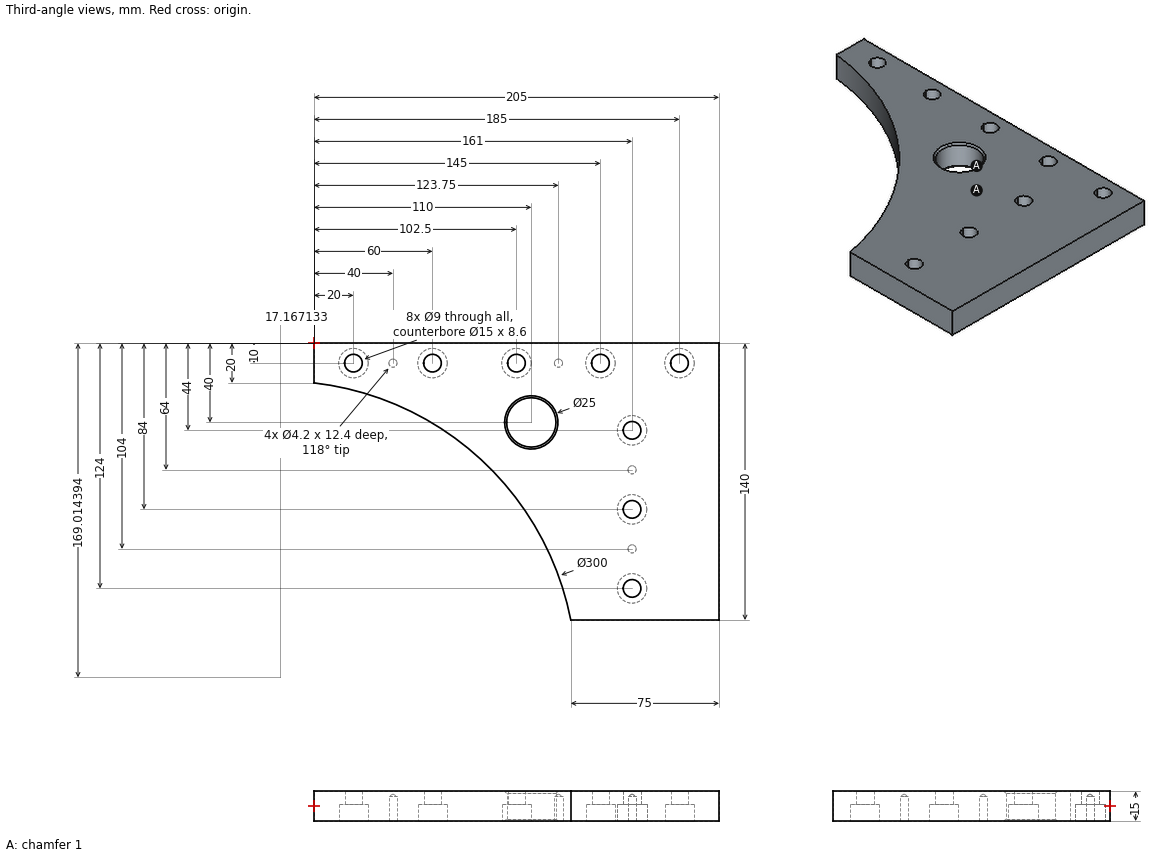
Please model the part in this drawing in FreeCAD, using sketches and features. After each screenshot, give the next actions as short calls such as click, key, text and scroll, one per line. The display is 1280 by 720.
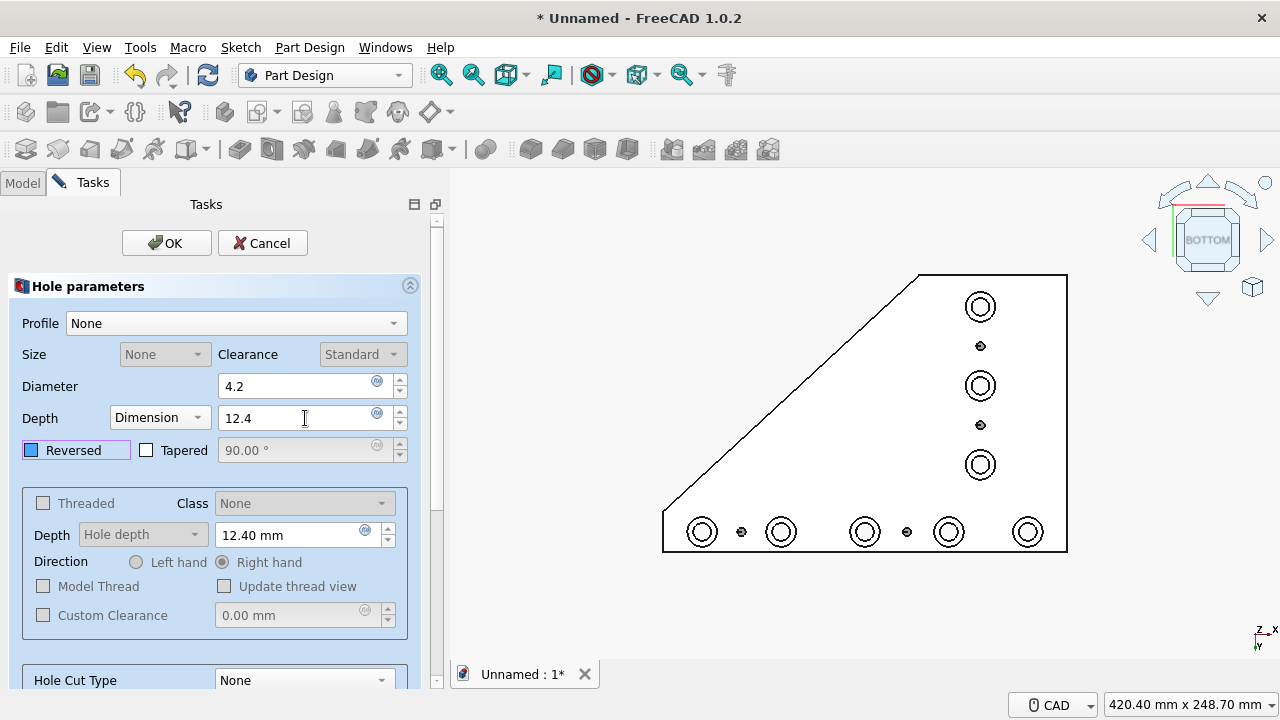
click(167, 243)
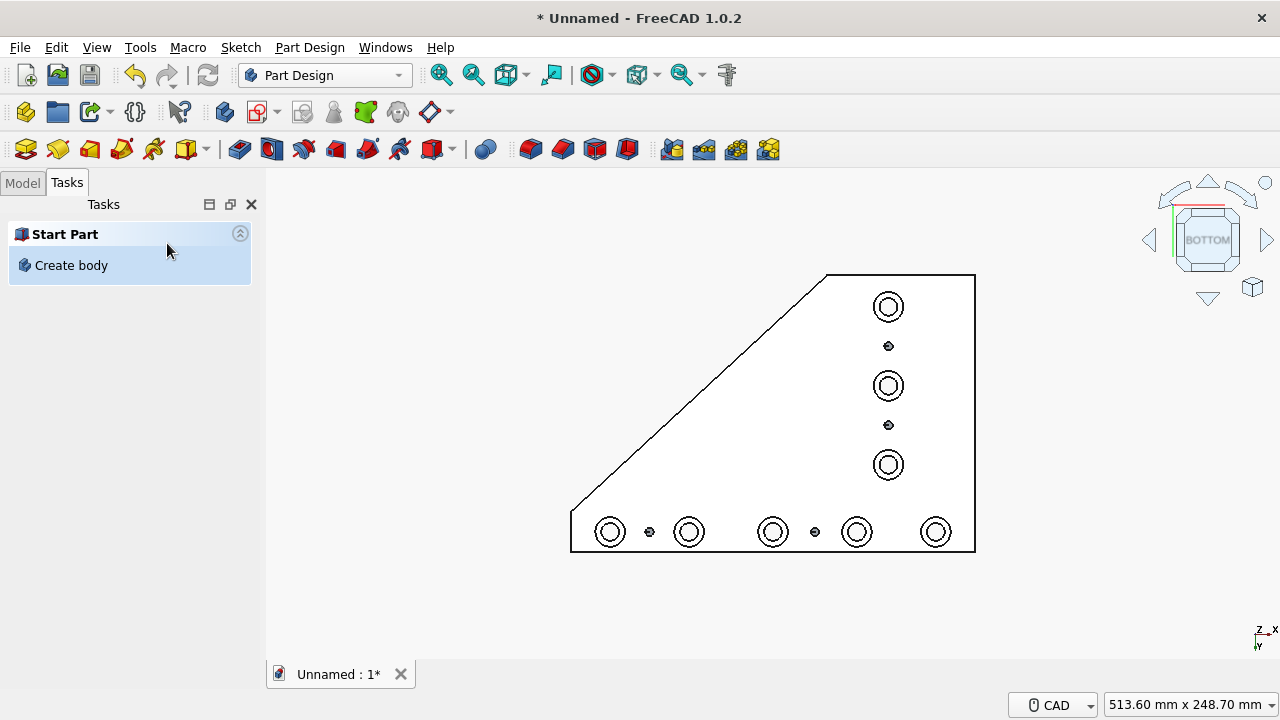
key(0)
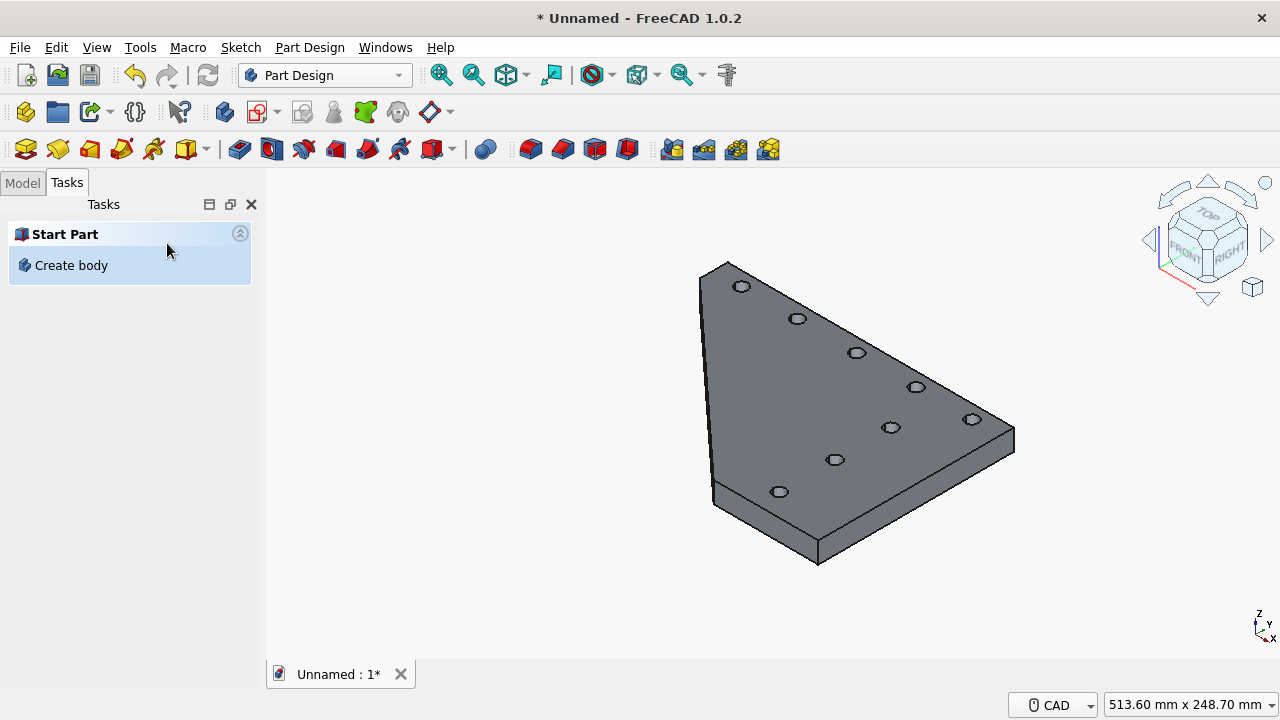
click(801, 384)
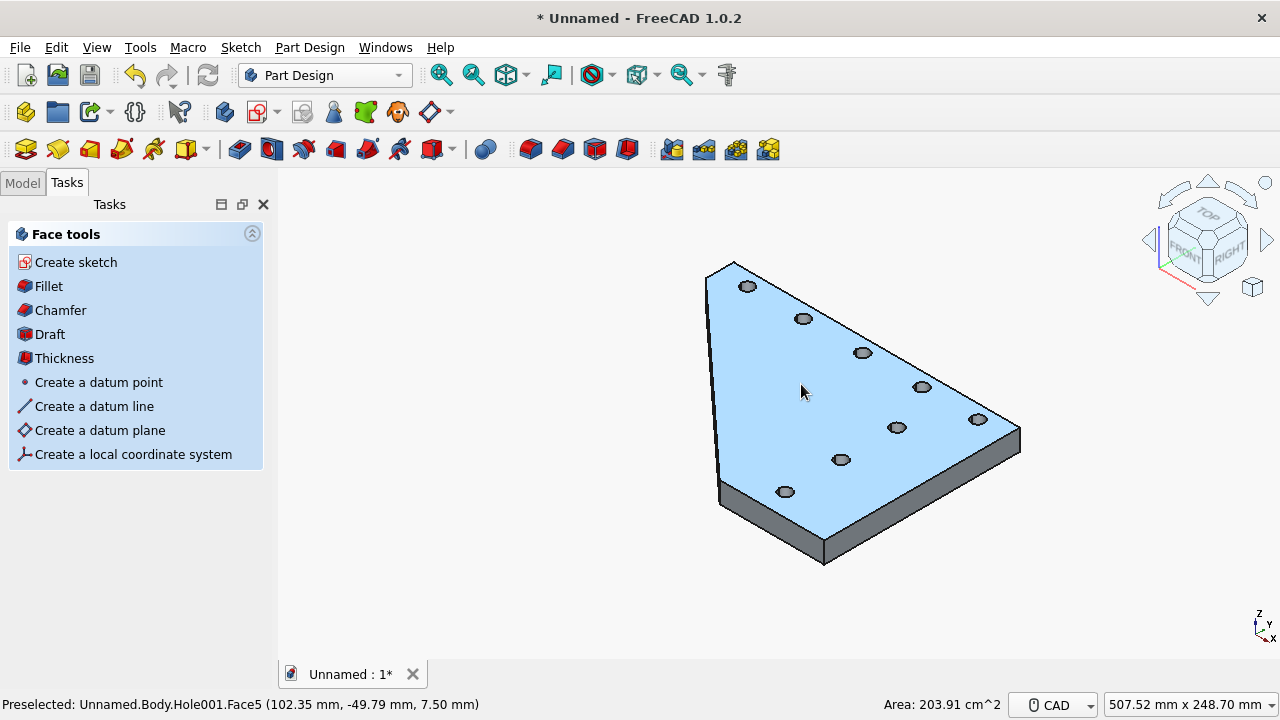
click(258, 112)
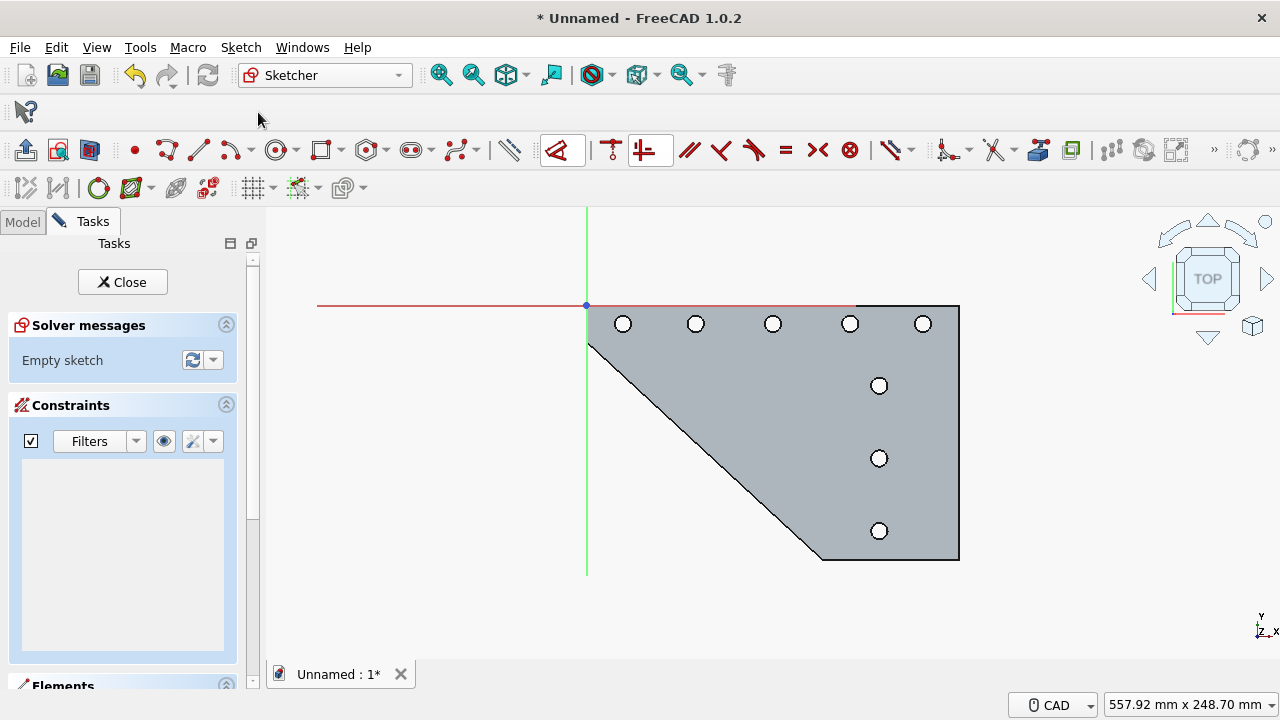
scroll(826, 300, down, 4)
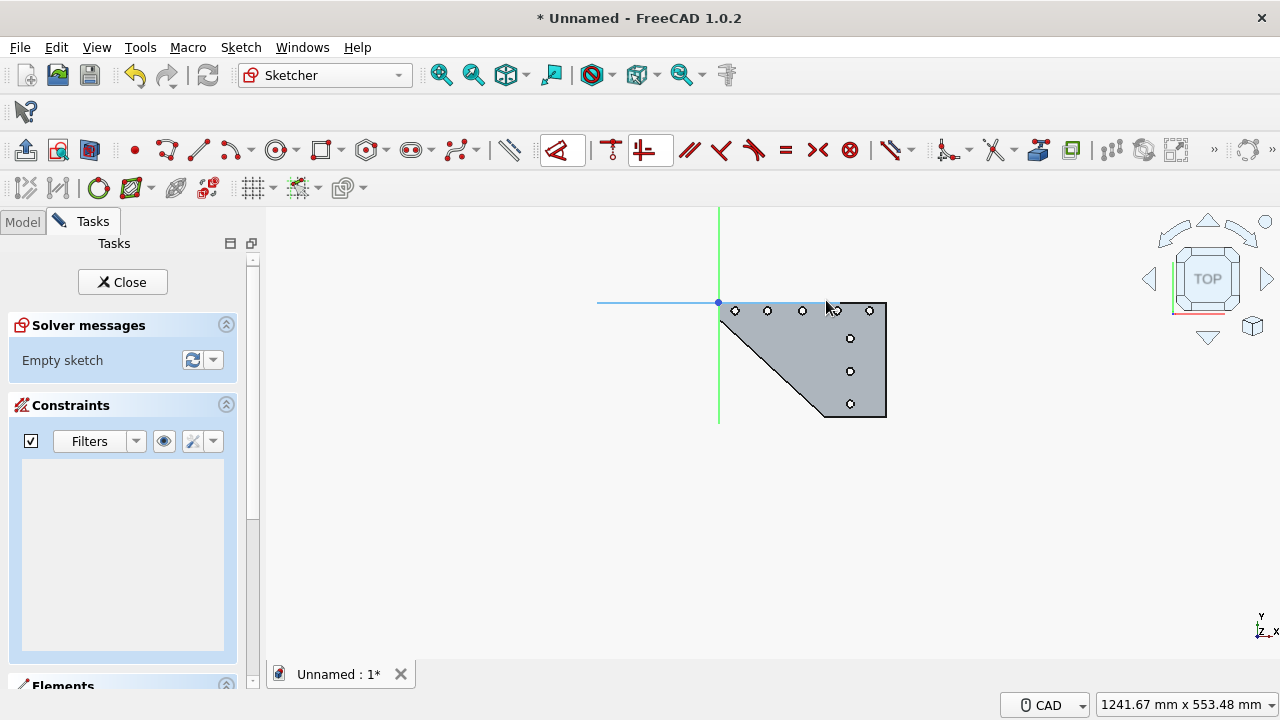
click(276, 150)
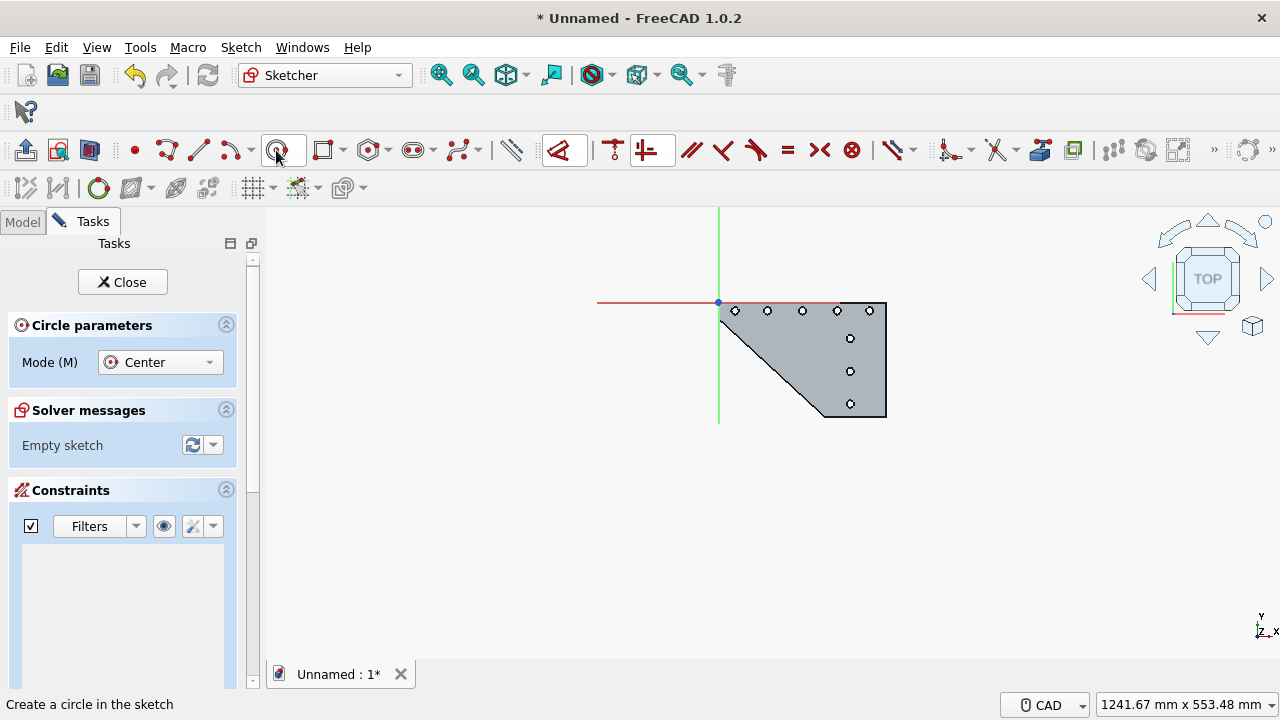
click(705, 441)
click(791, 354)
key(Escape)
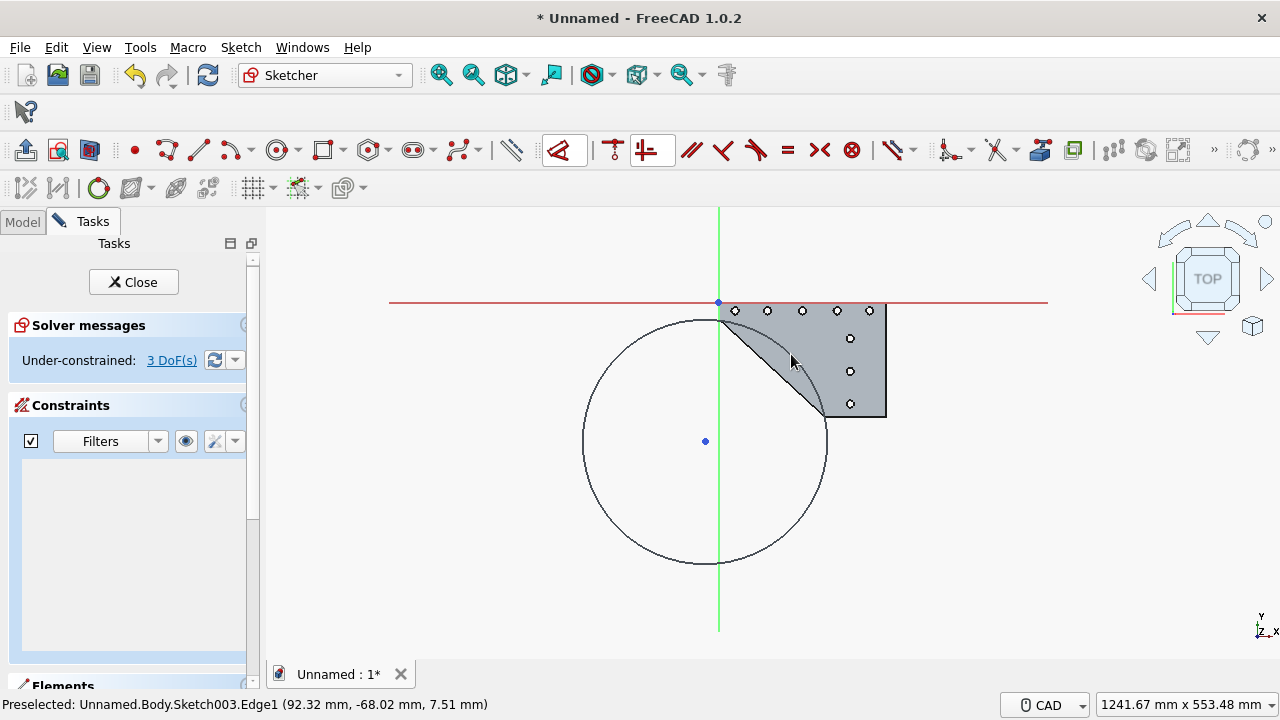
click(791, 355)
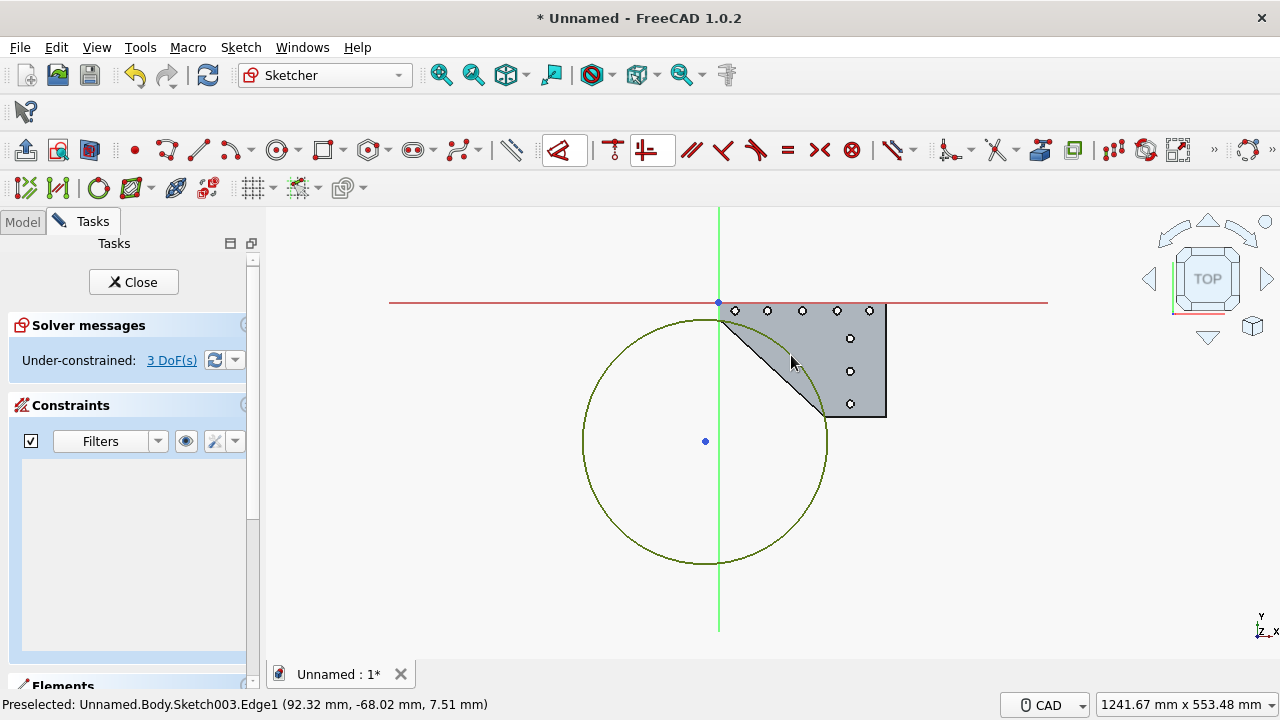
click(582, 150)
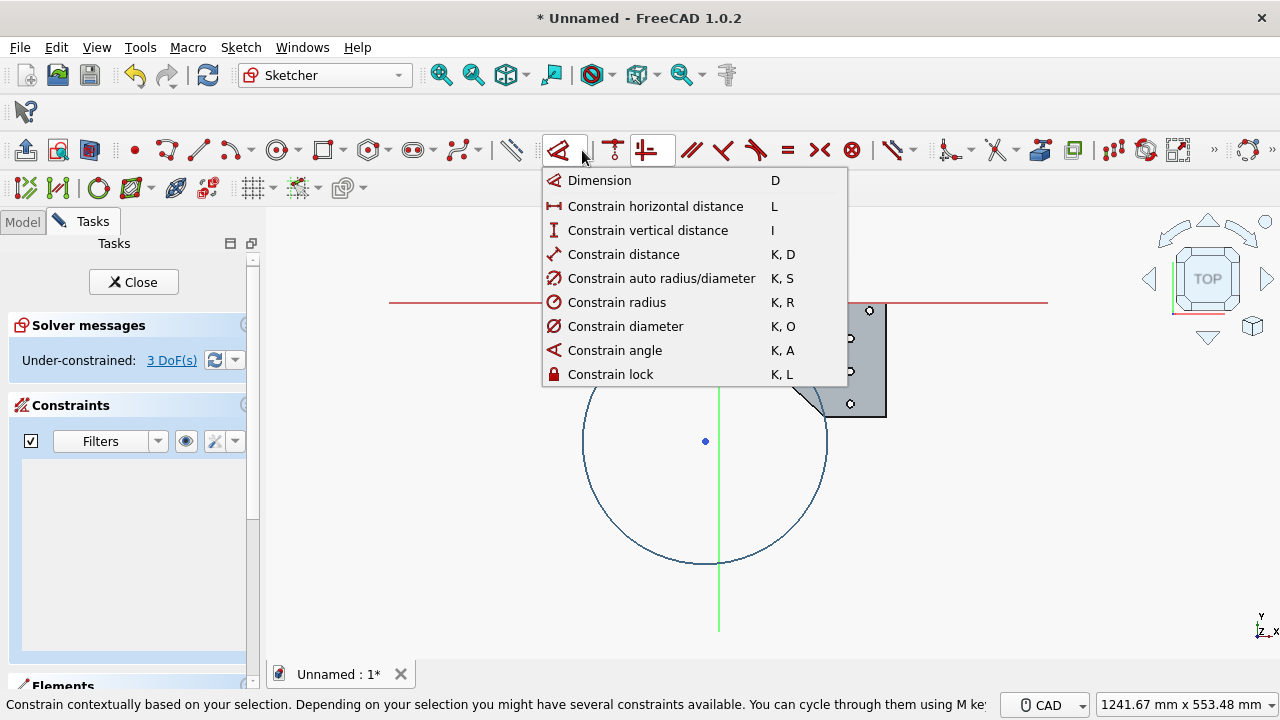
click(695, 326)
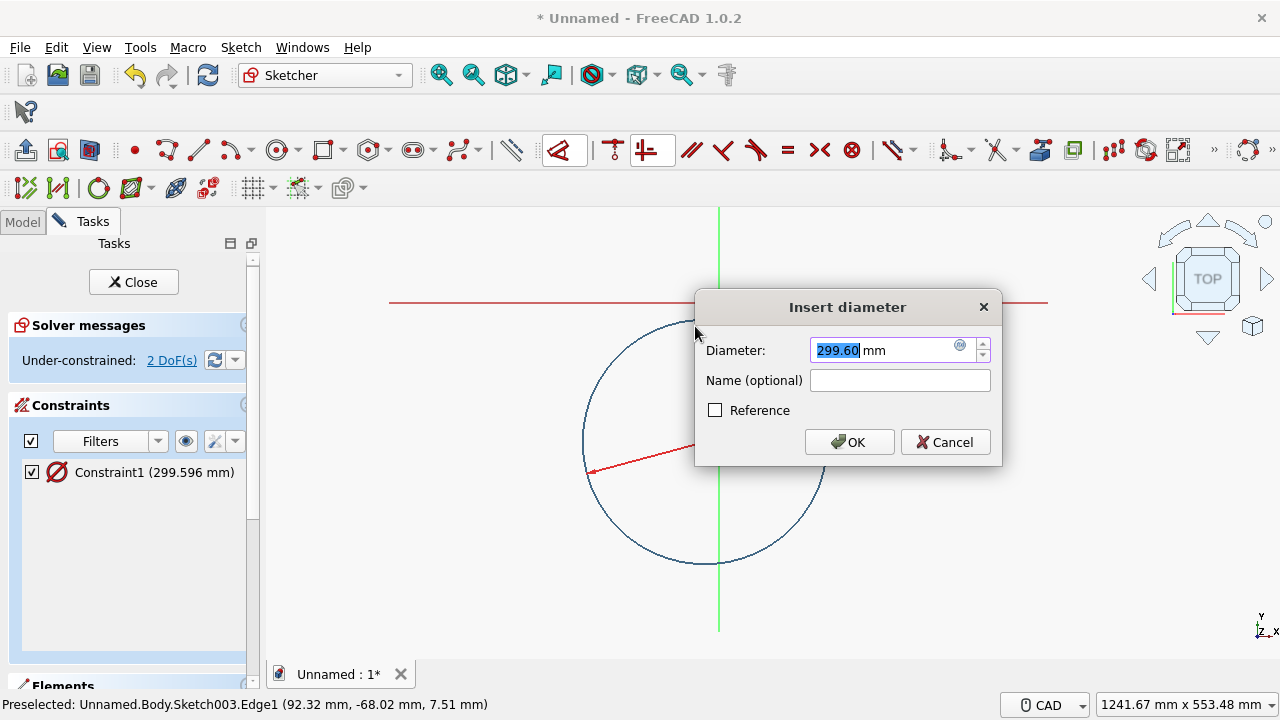
text(300)
key(Return)